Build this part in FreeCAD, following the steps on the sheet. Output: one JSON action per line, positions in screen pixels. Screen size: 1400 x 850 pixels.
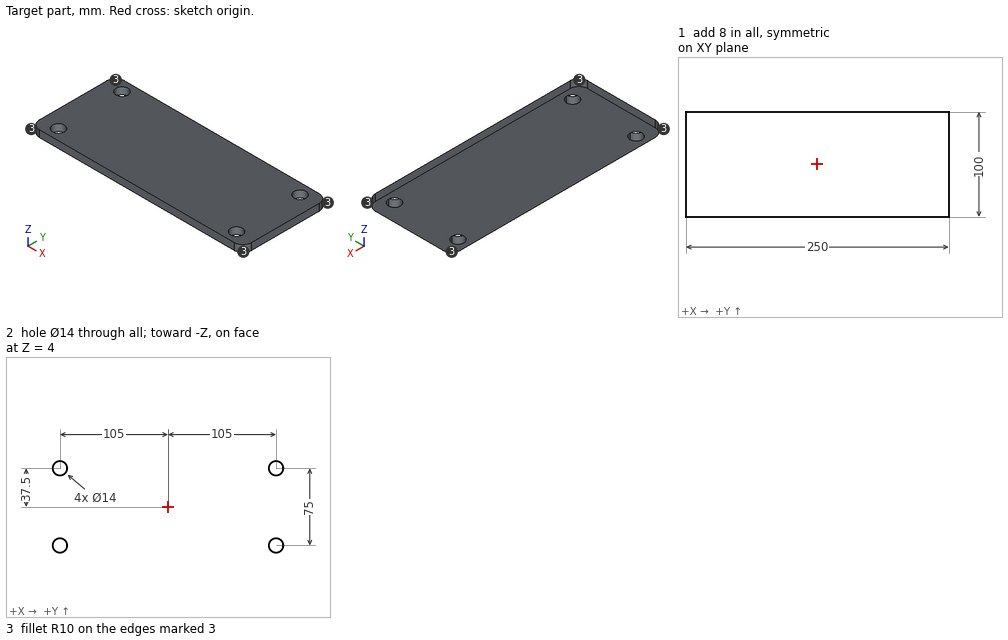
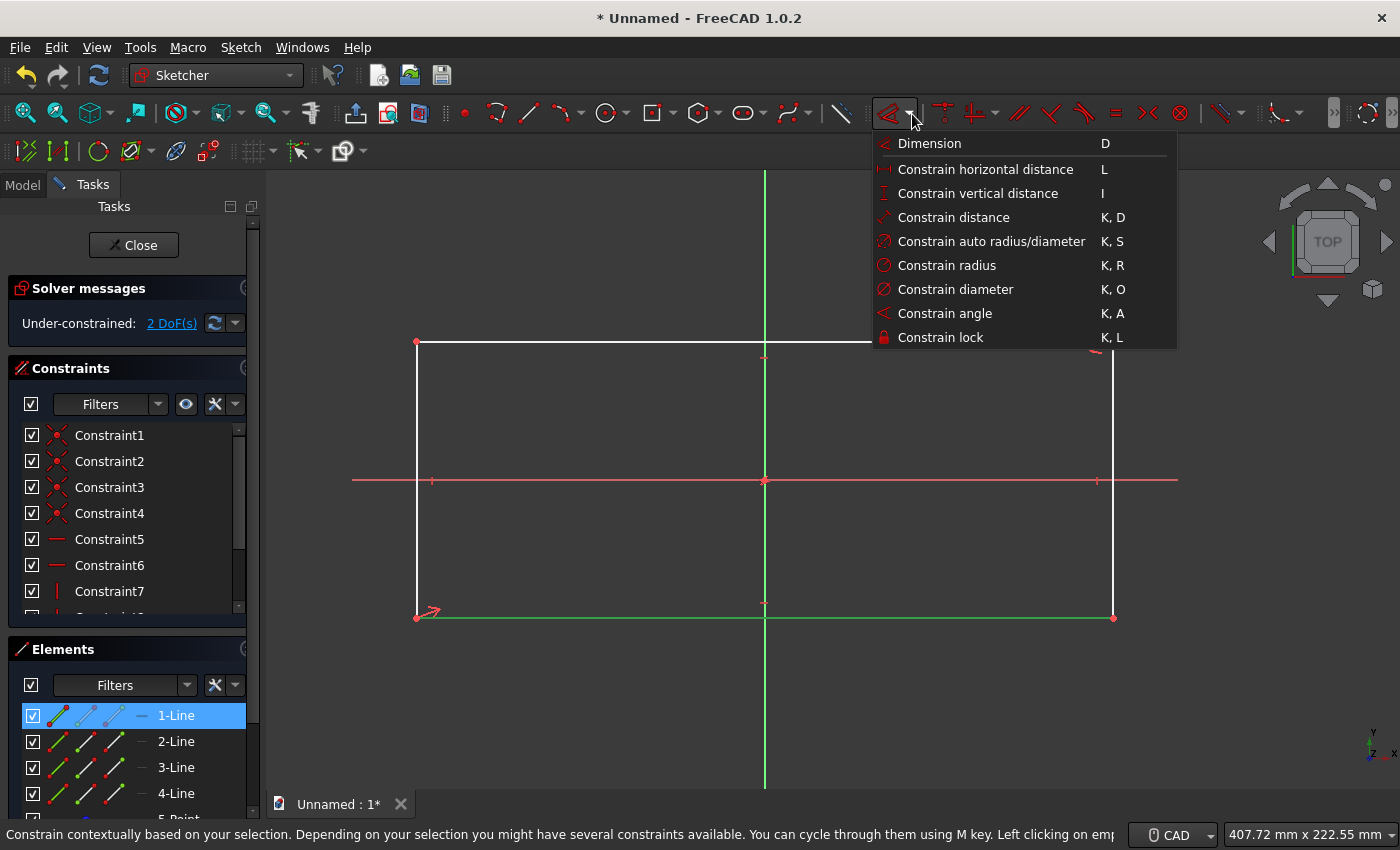
{"action": "left_click", "coordinate": [1025, 169]}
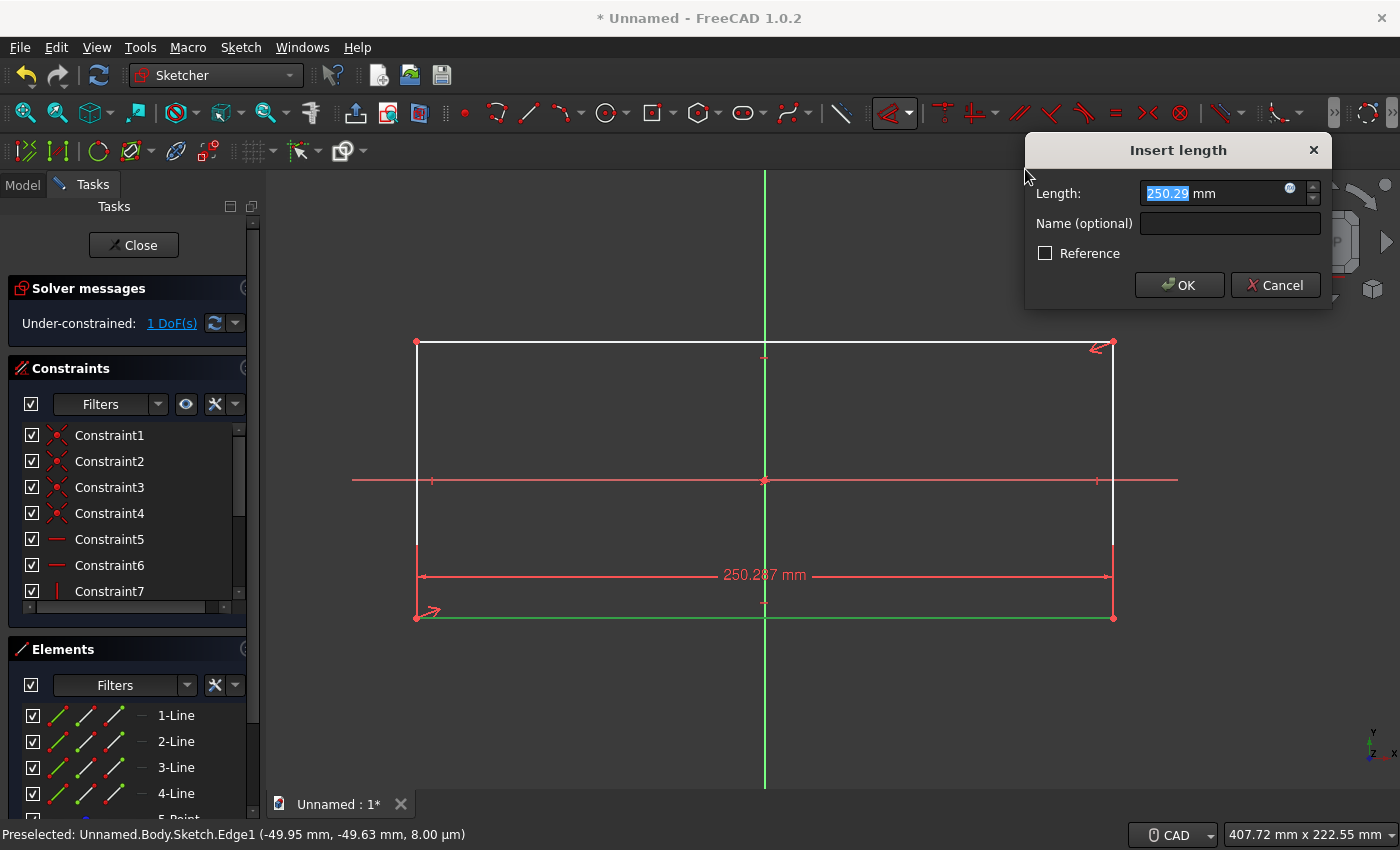
{"action": "type", "text": "250"}
{"action": "key", "text": "Return"}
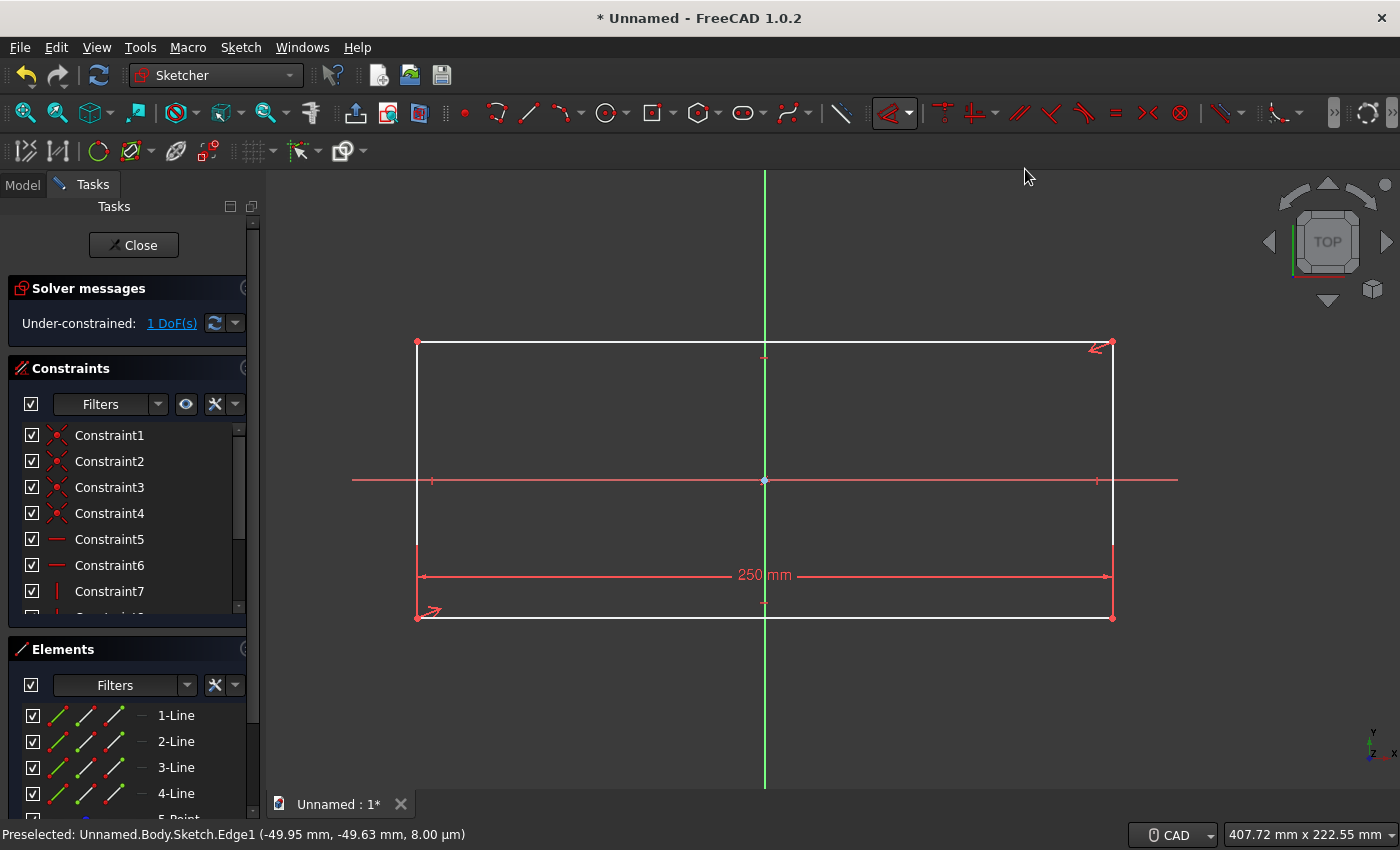
{"action": "left_click", "coordinate": [1113, 535]}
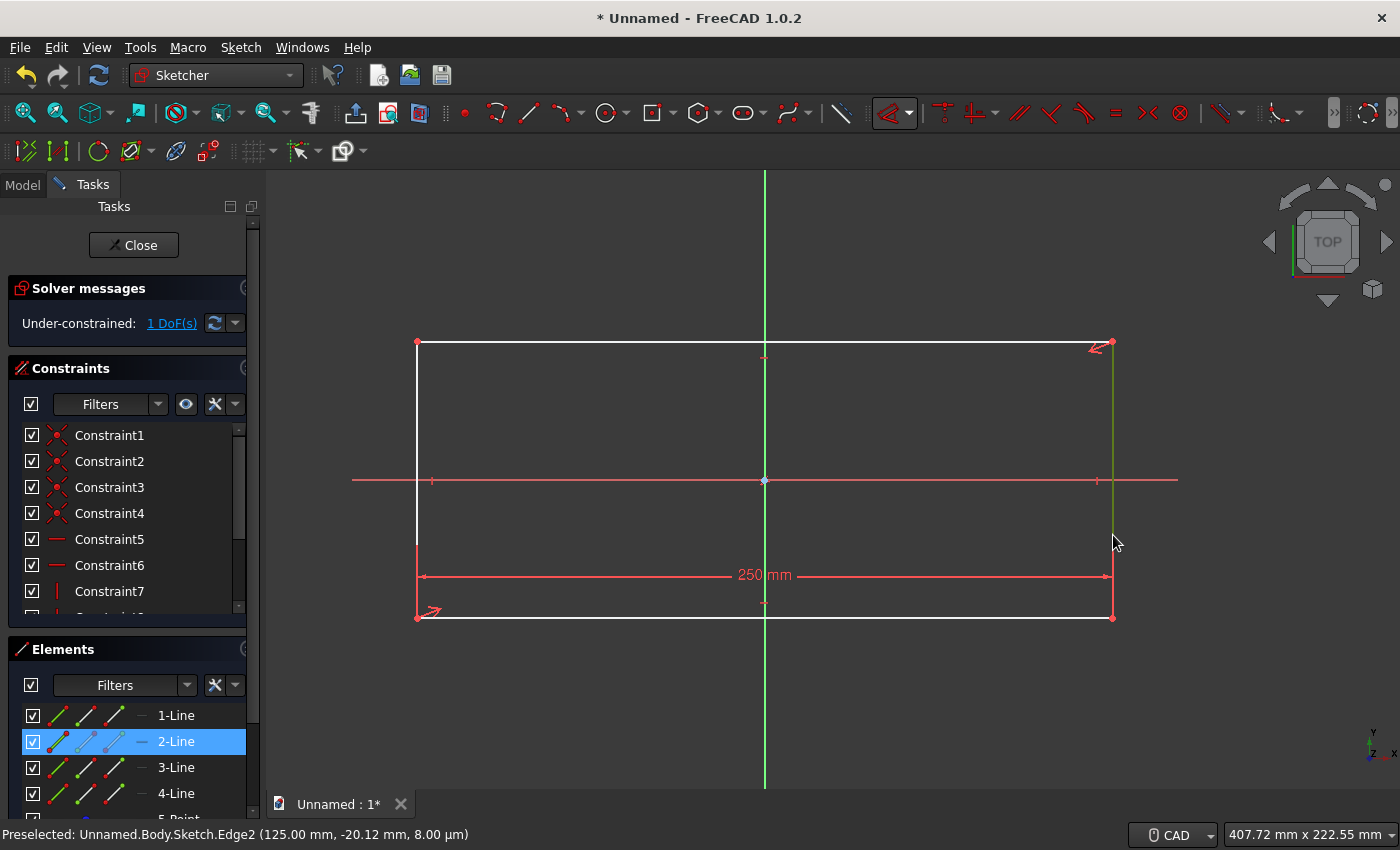
{"action": "left_click", "coordinate": [912, 114]}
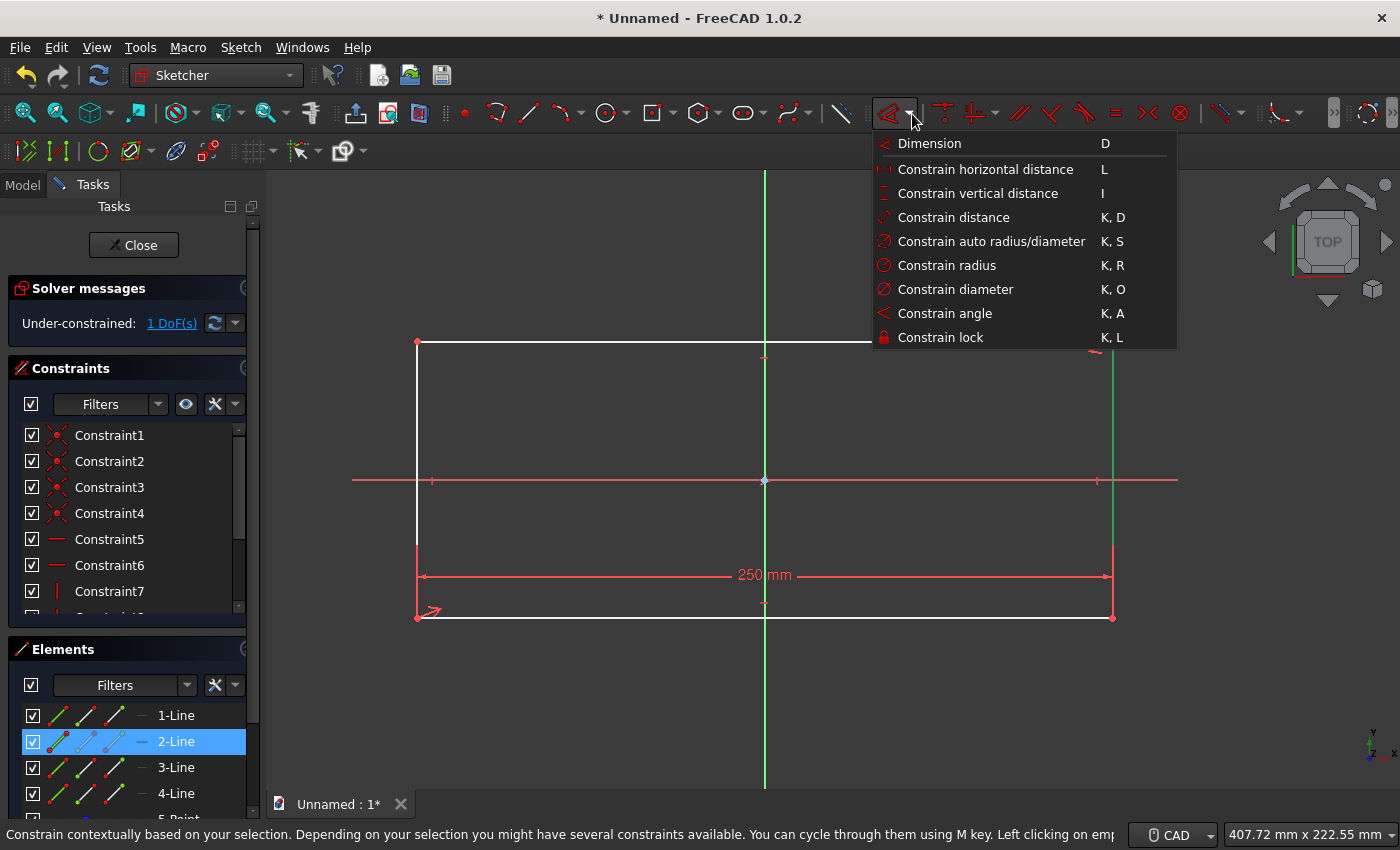
{"action": "left_click", "coordinate": [1025, 193]}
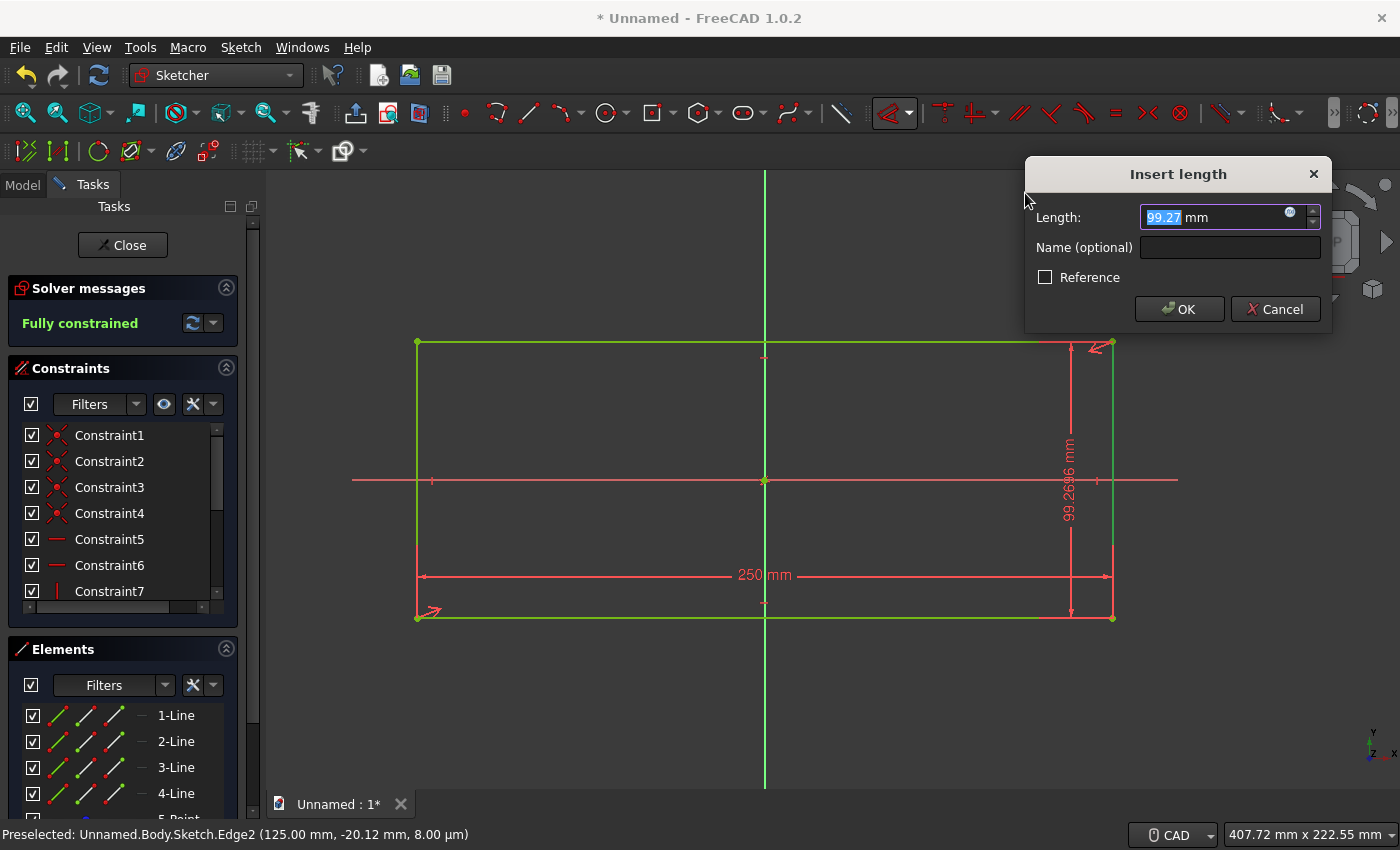
{"action": "type", "text": "100"}
{"action": "key", "text": "Return"}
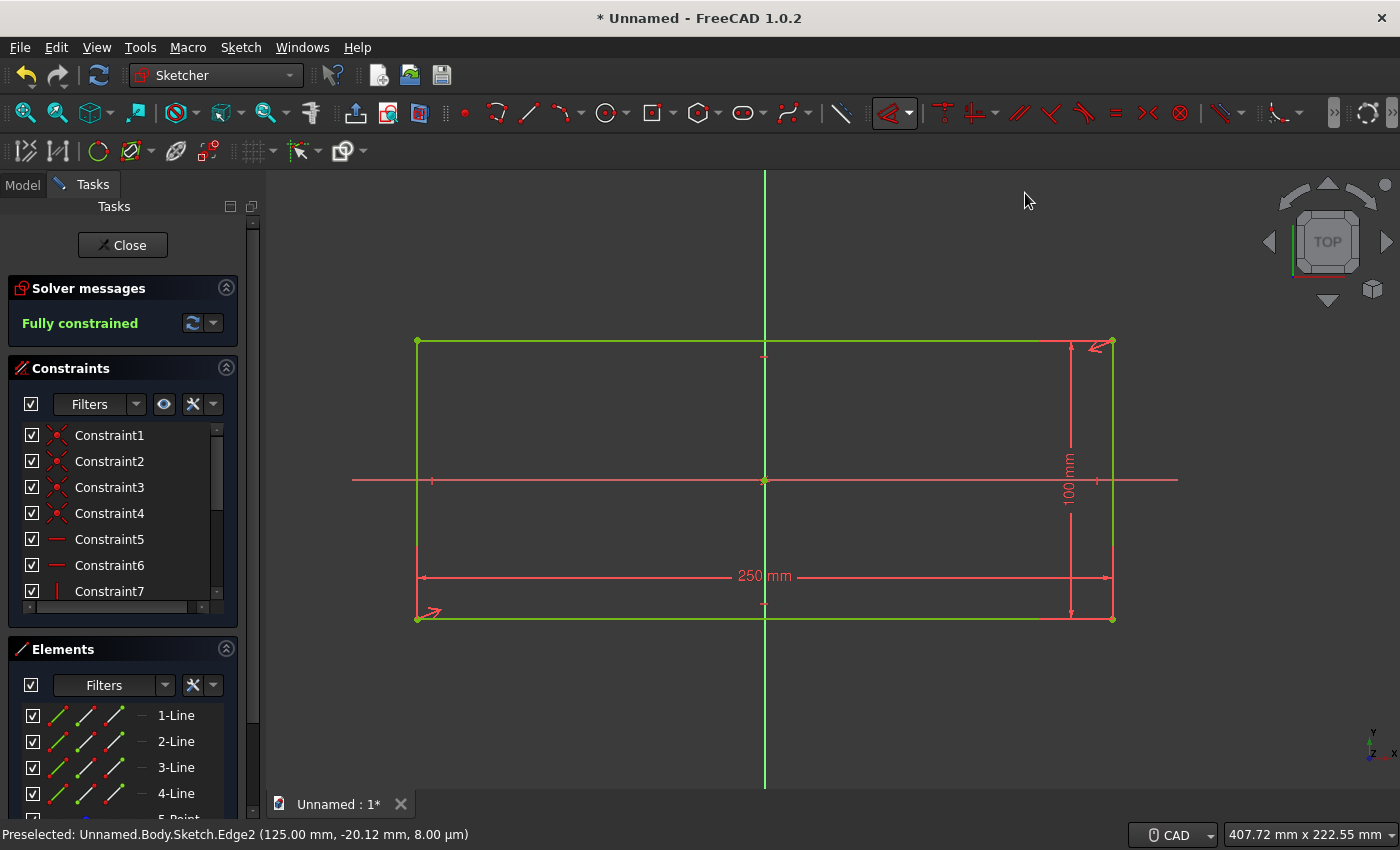
{"action": "left_click", "coordinate": [123, 245]}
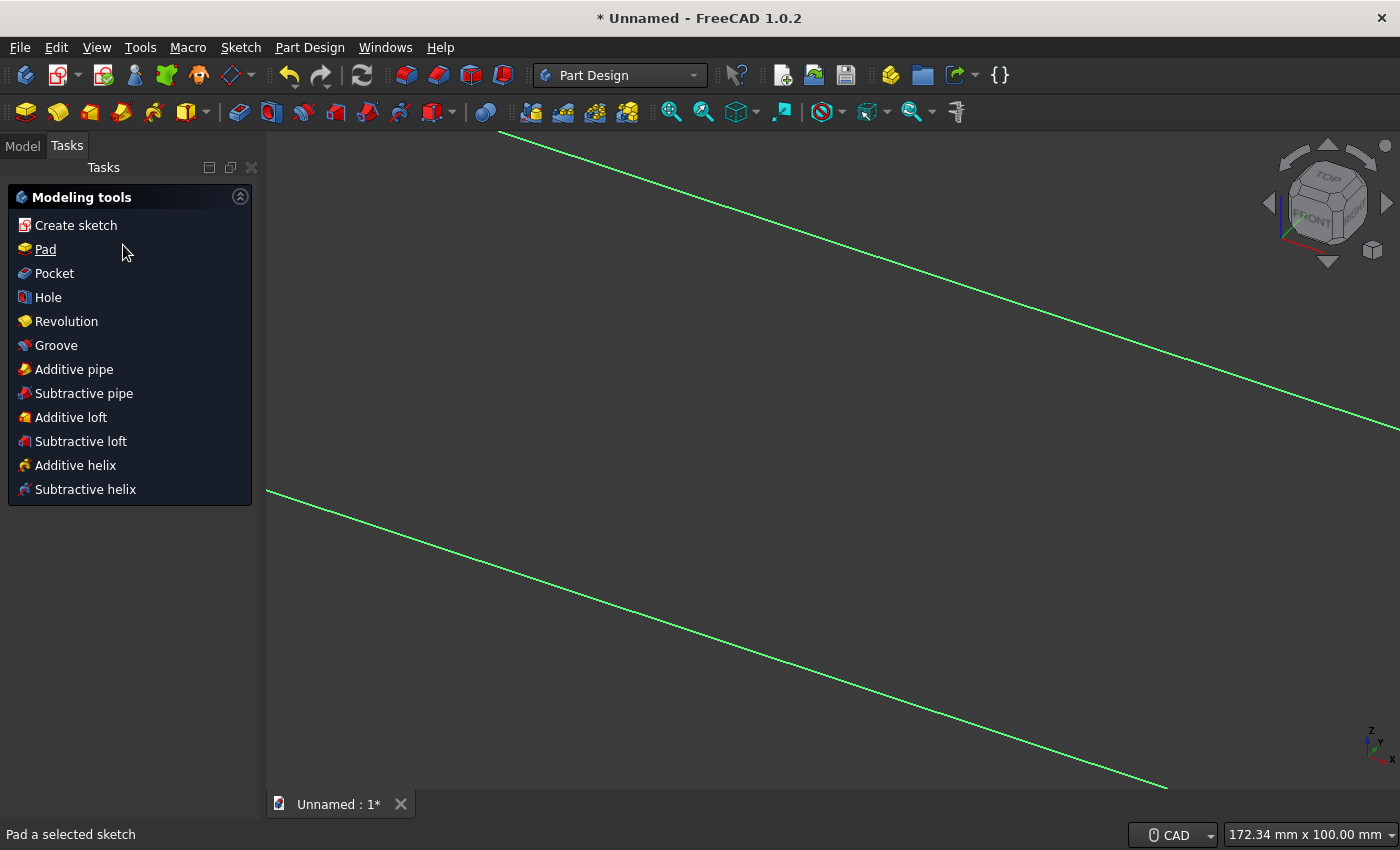
{"action": "left_click", "coordinate": [26, 112]}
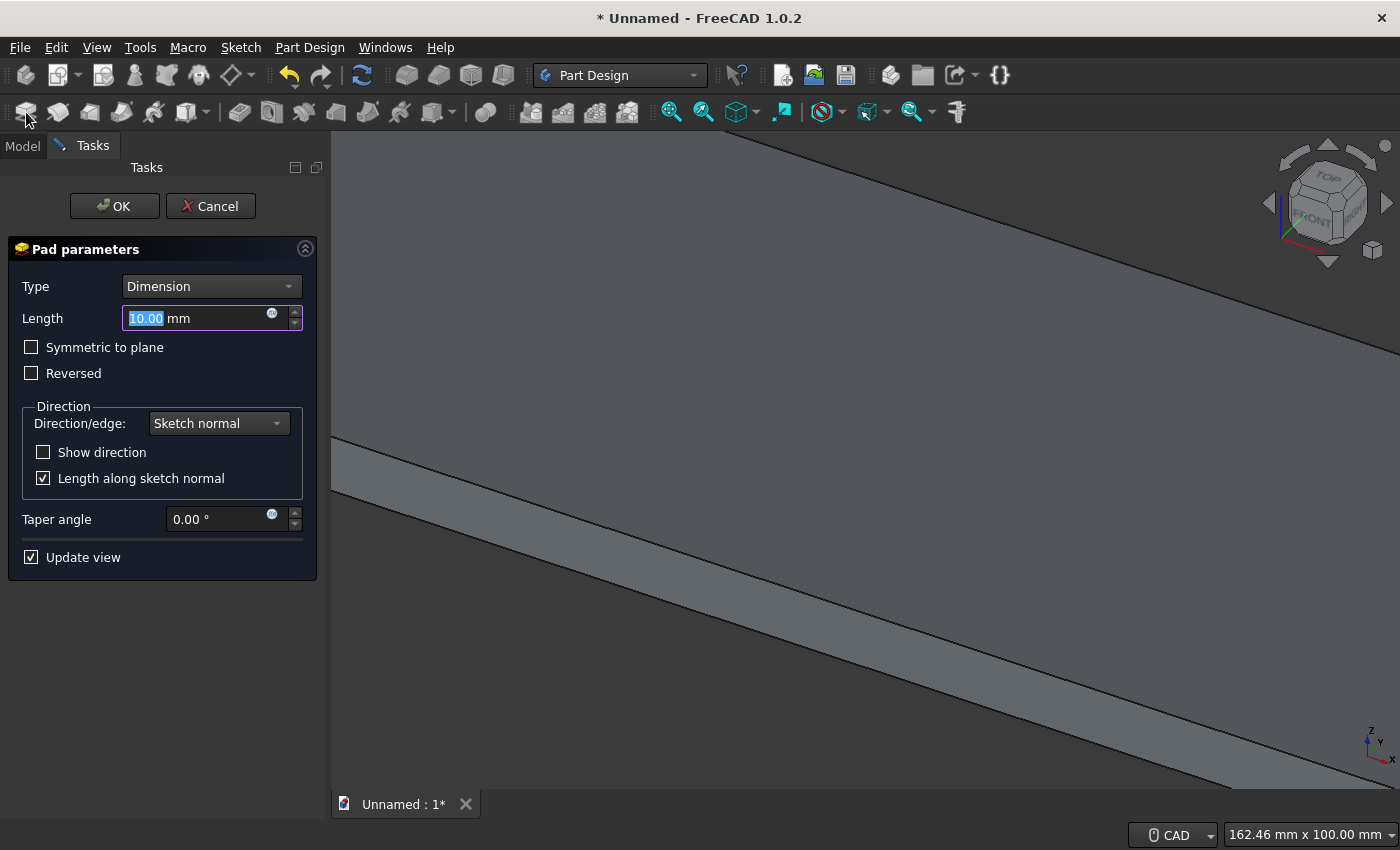
{"action": "type", "text": "8"}
{"action": "key", "text": "Tab"}